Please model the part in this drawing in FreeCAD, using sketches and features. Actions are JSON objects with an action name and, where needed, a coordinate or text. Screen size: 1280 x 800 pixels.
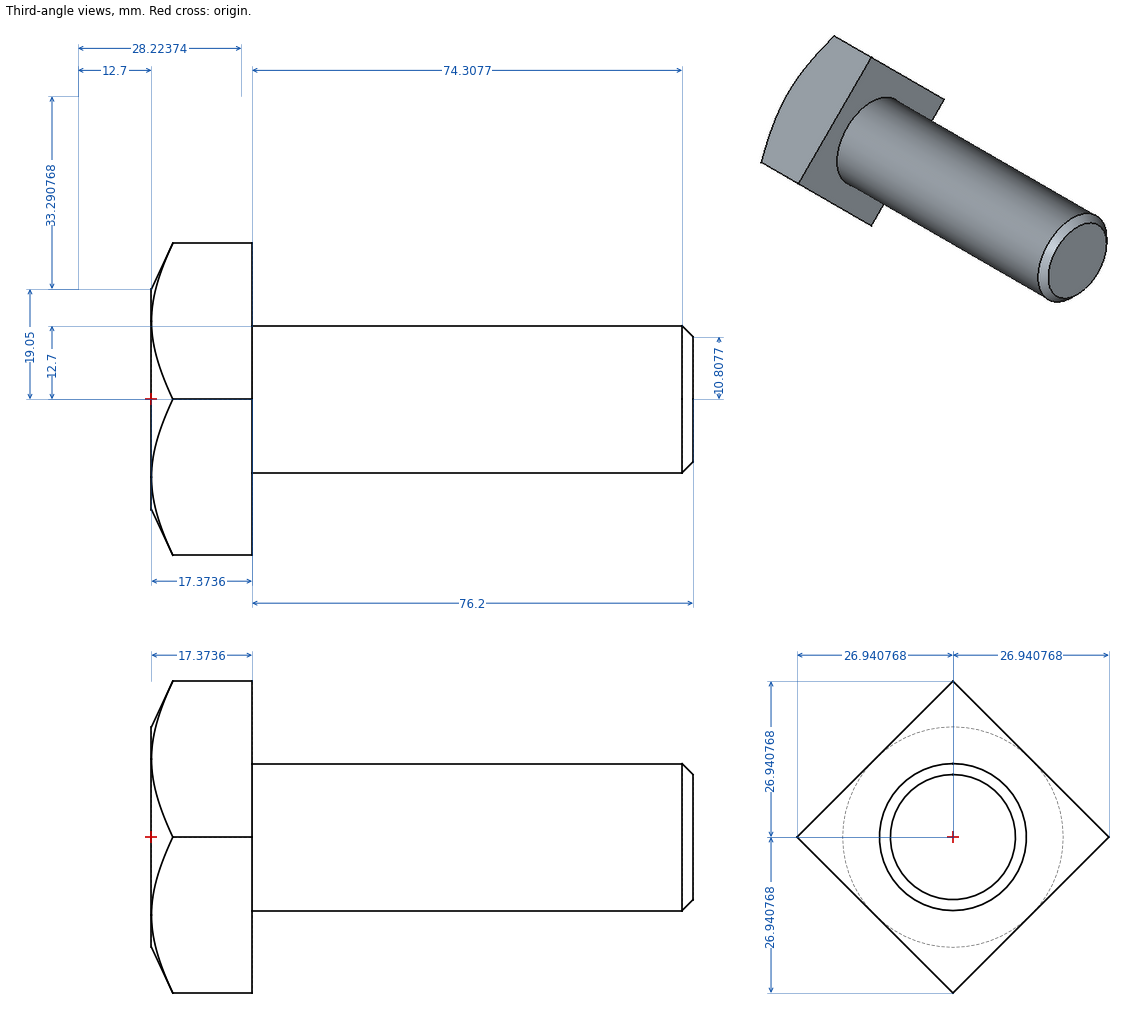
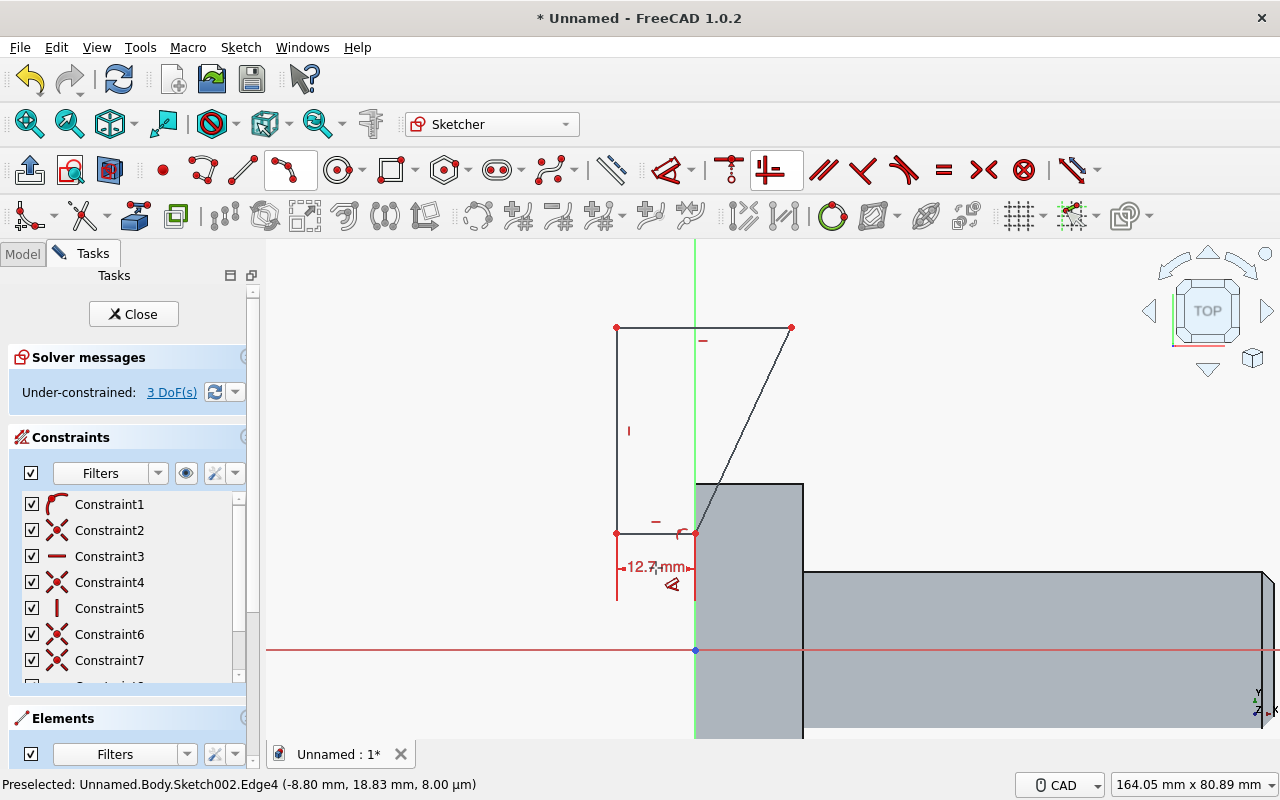
{"action": "left_click", "coordinate": [695, 534]}
{"action": "left_click", "coordinate": [661, 592]}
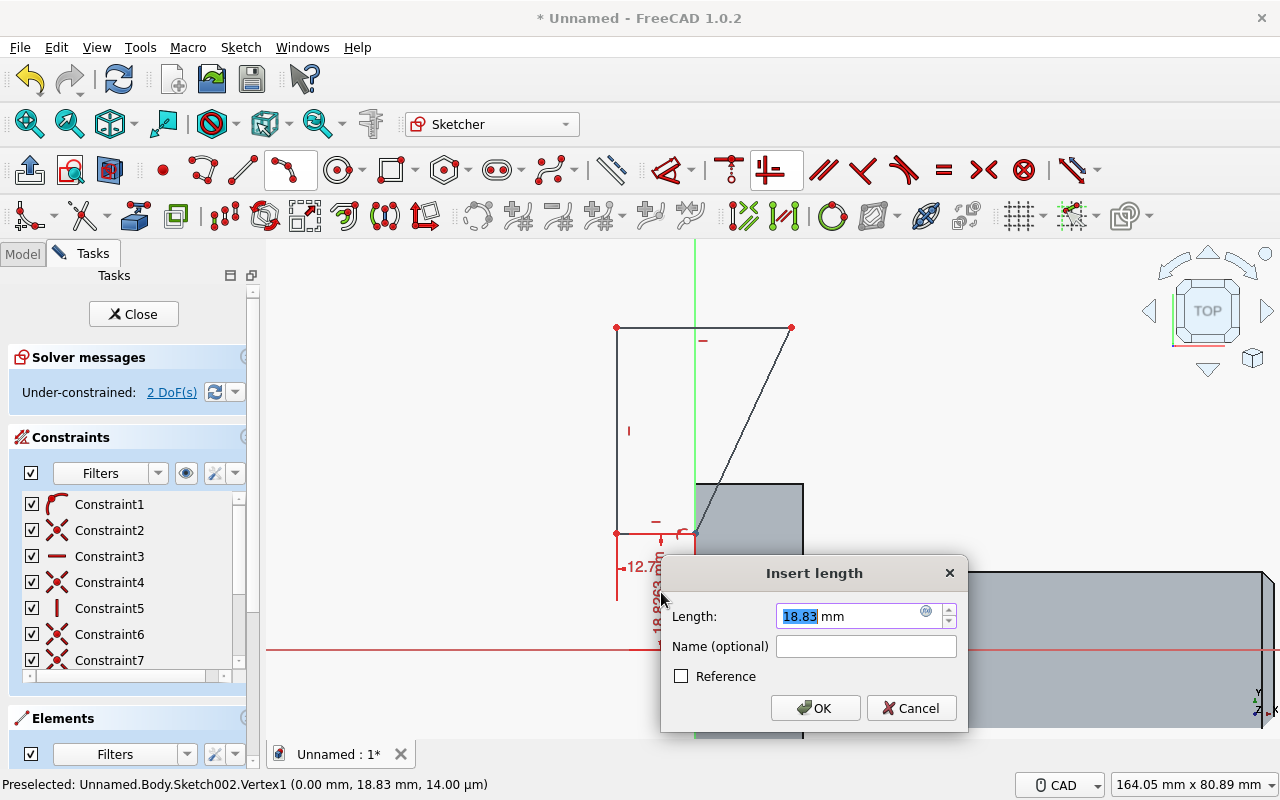
{"action": "type", "text": "19.05"}
{"action": "key", "text": "Return"}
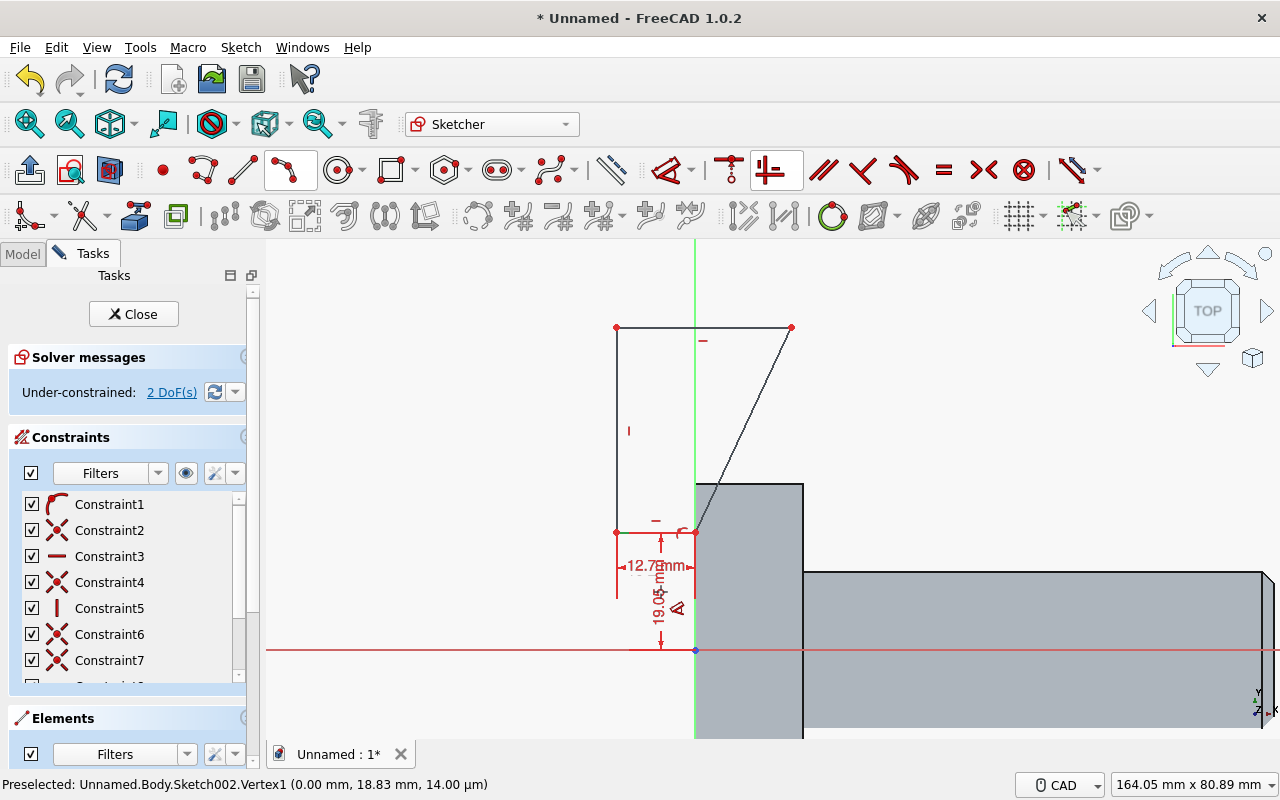
{"action": "left_click", "coordinate": [739, 328]}
{"action": "left_click", "coordinate": [664, 294]}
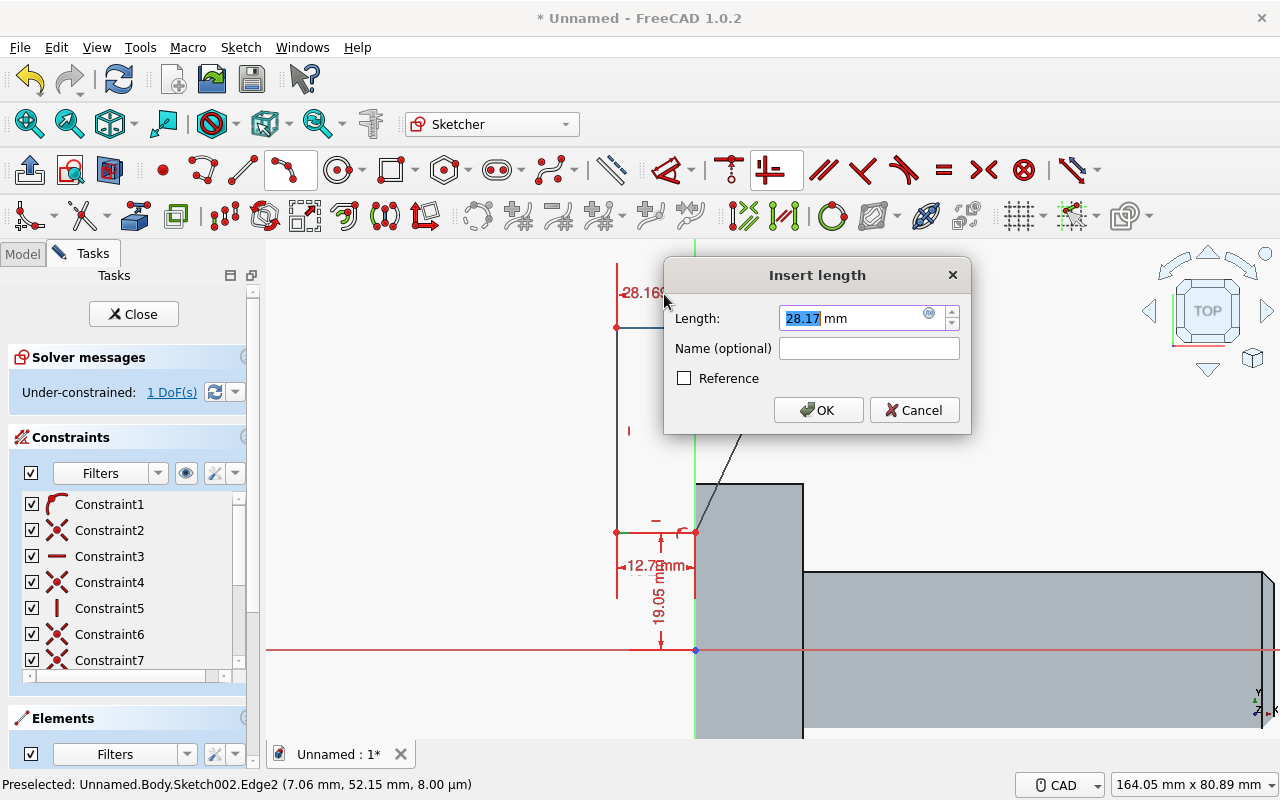
{"action": "type", "text": "28.22374"}
{"action": "key", "text": "Return"}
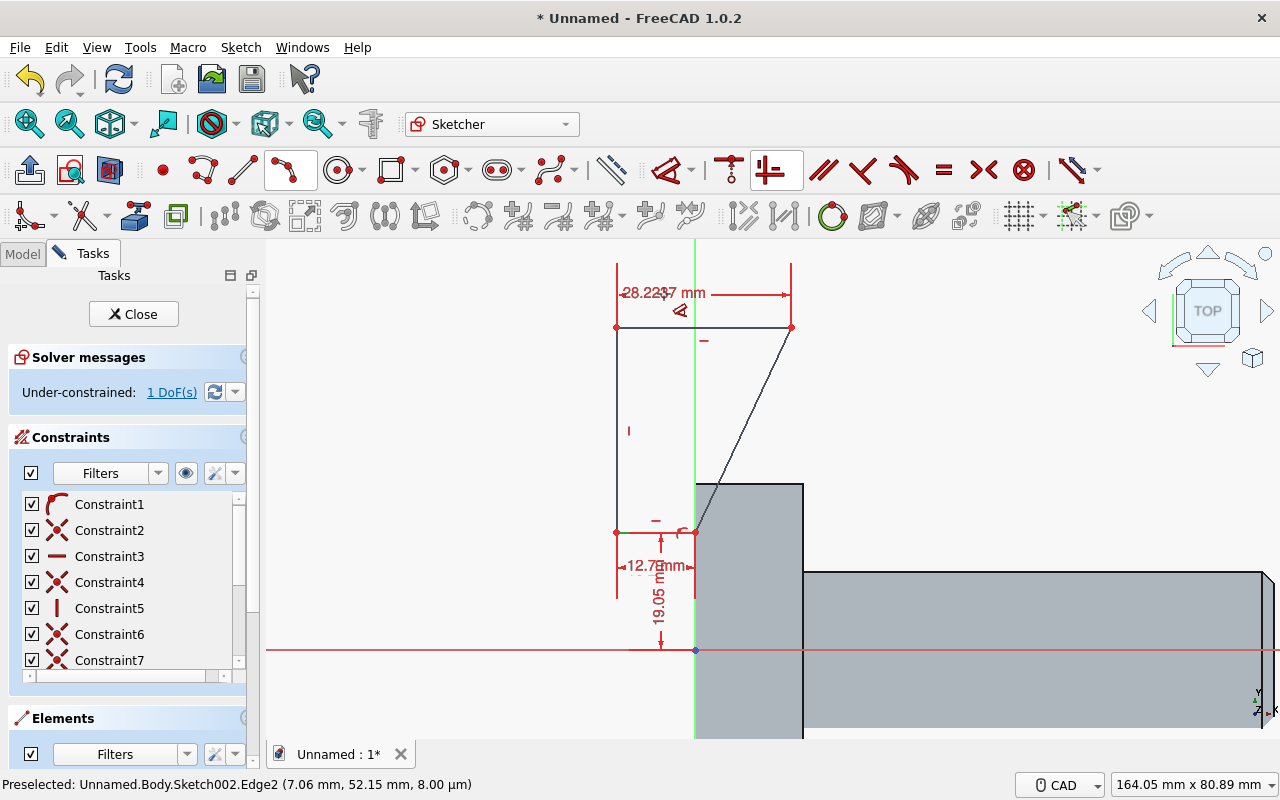
{"action": "left_click", "coordinate": [617, 389]}
{"action": "left_click", "coordinate": [583, 430]}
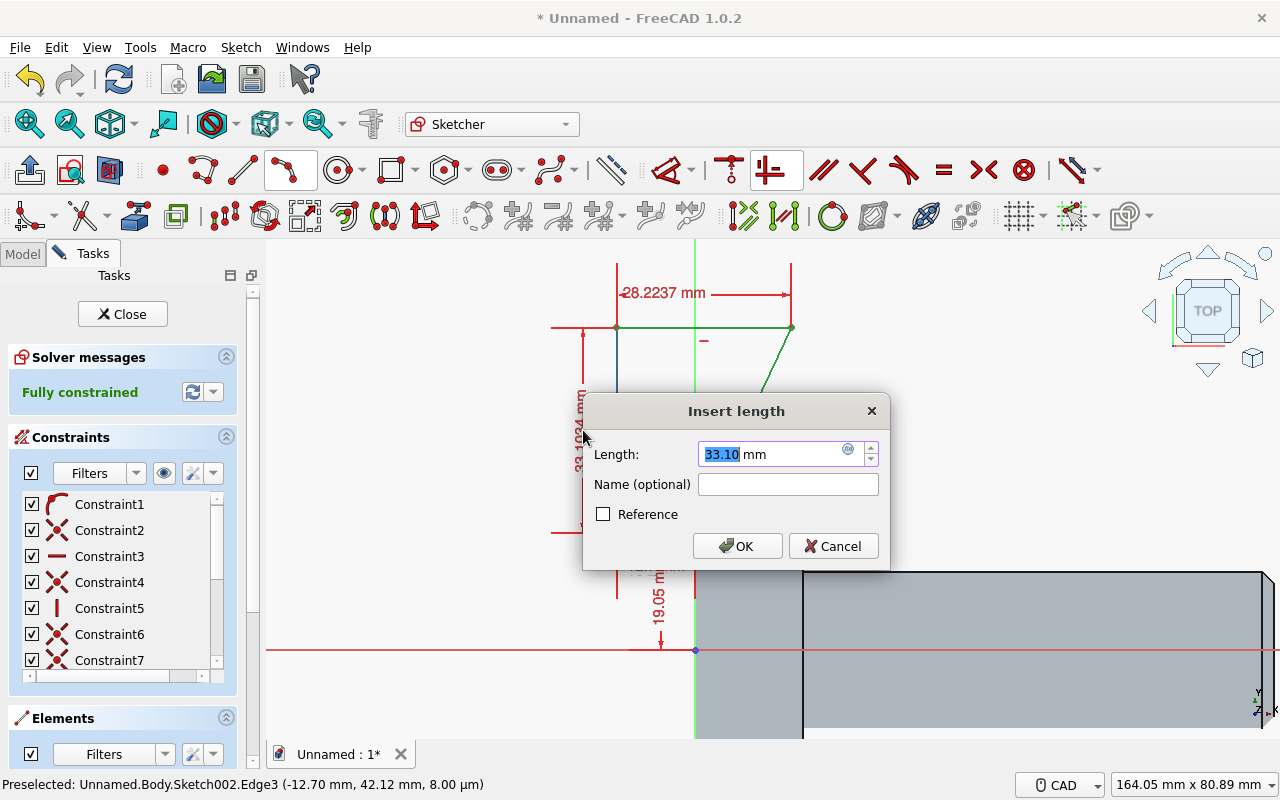
{"action": "type", "text": "33.290768"}
{"action": "key", "text": "Return"}
{"action": "key", "text": "Escape"}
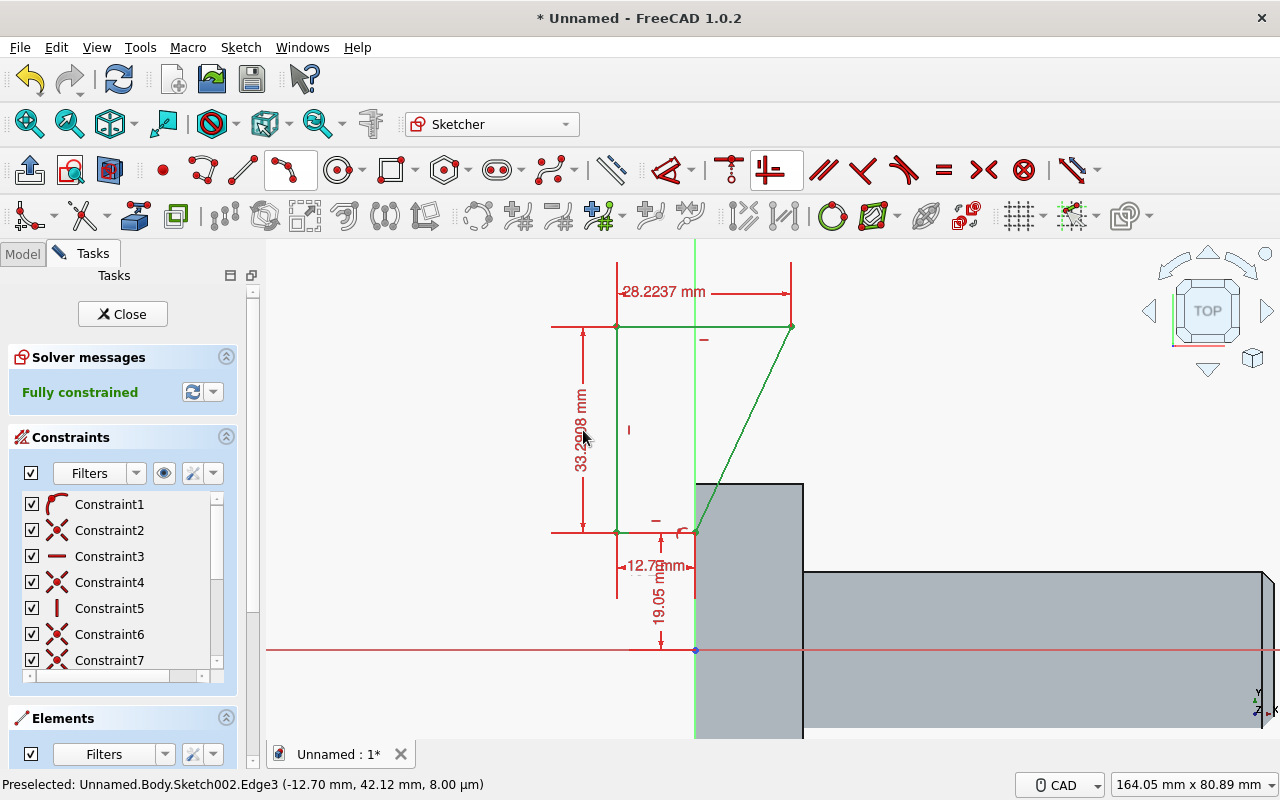
{"action": "left_click", "coordinate": [123, 314]}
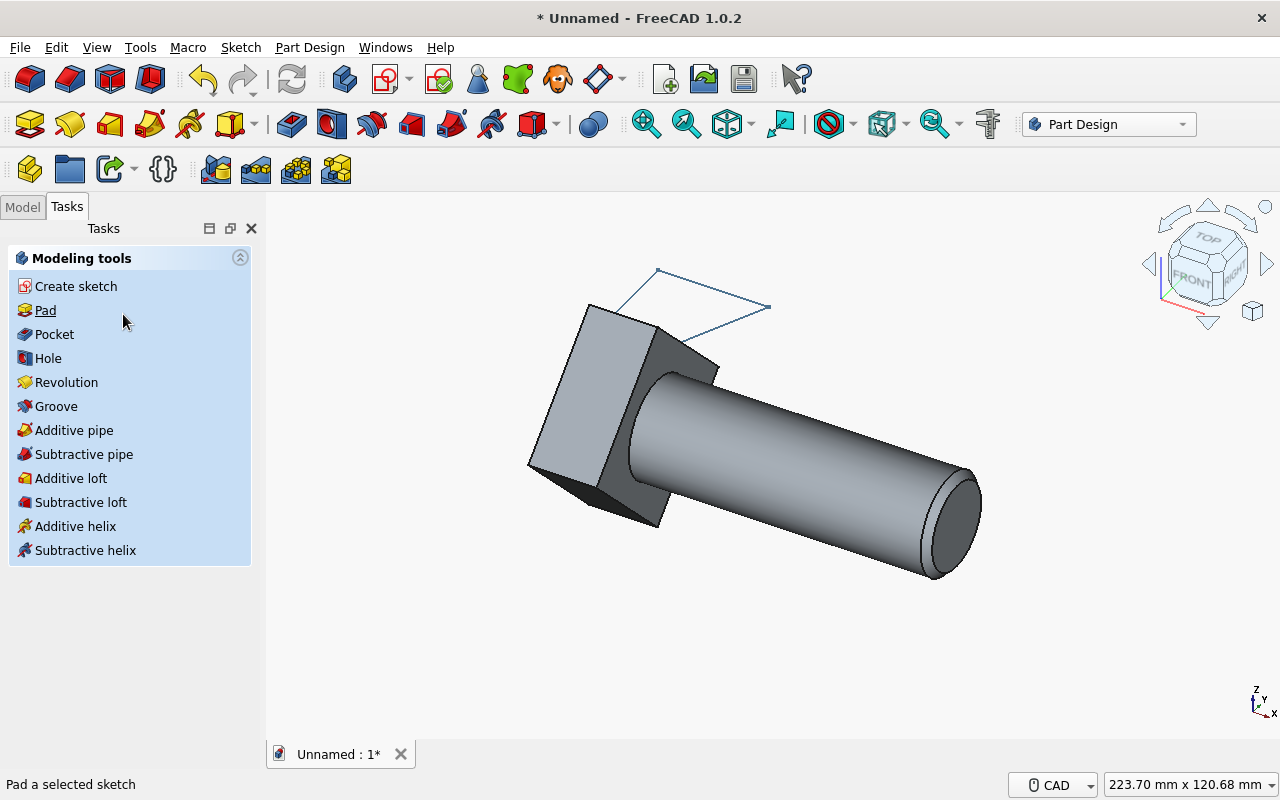
{"action": "left_click", "coordinate": [372, 124]}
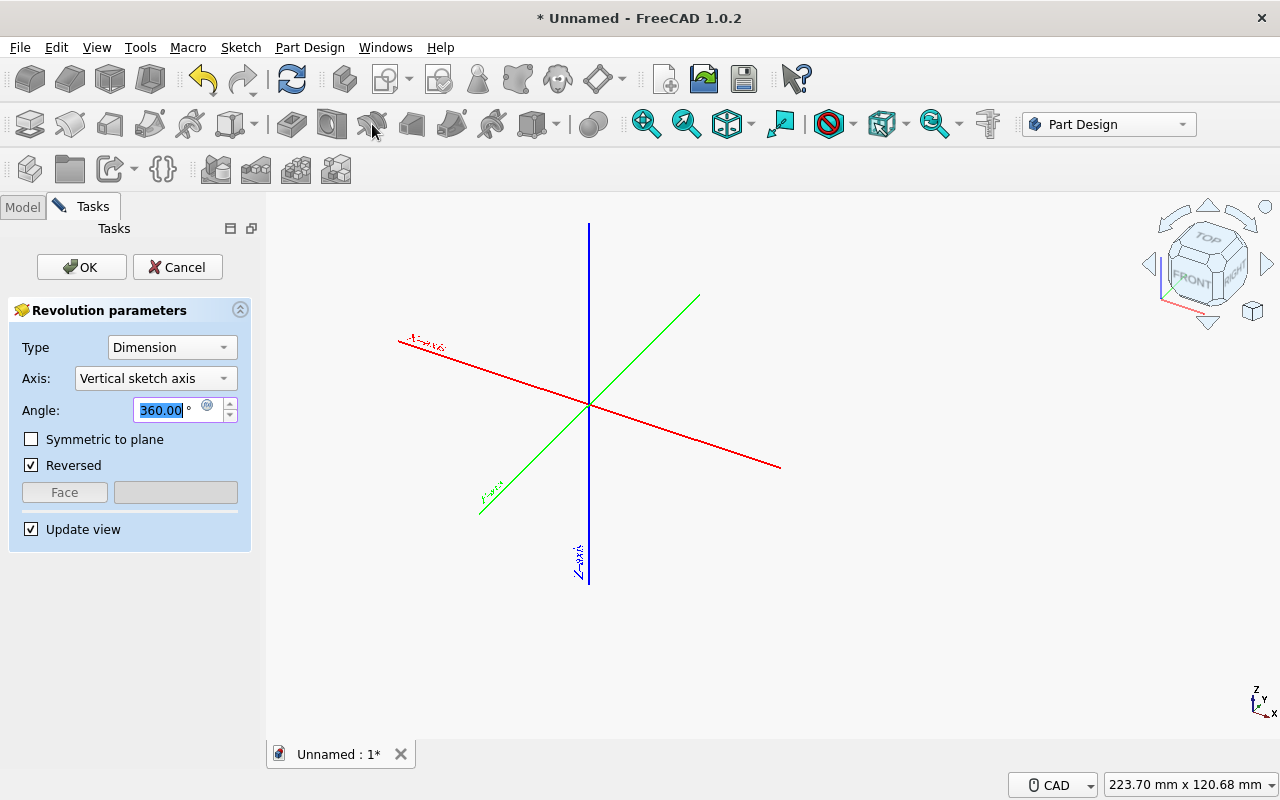
{"action": "left_click", "coordinate": [156, 378]}